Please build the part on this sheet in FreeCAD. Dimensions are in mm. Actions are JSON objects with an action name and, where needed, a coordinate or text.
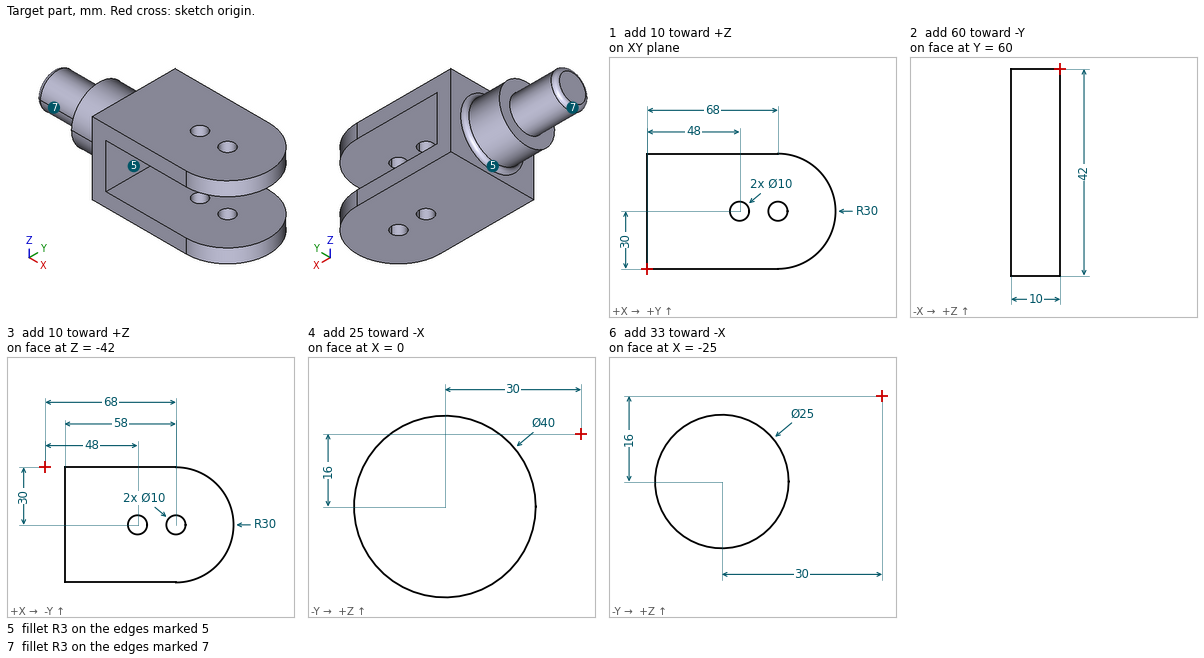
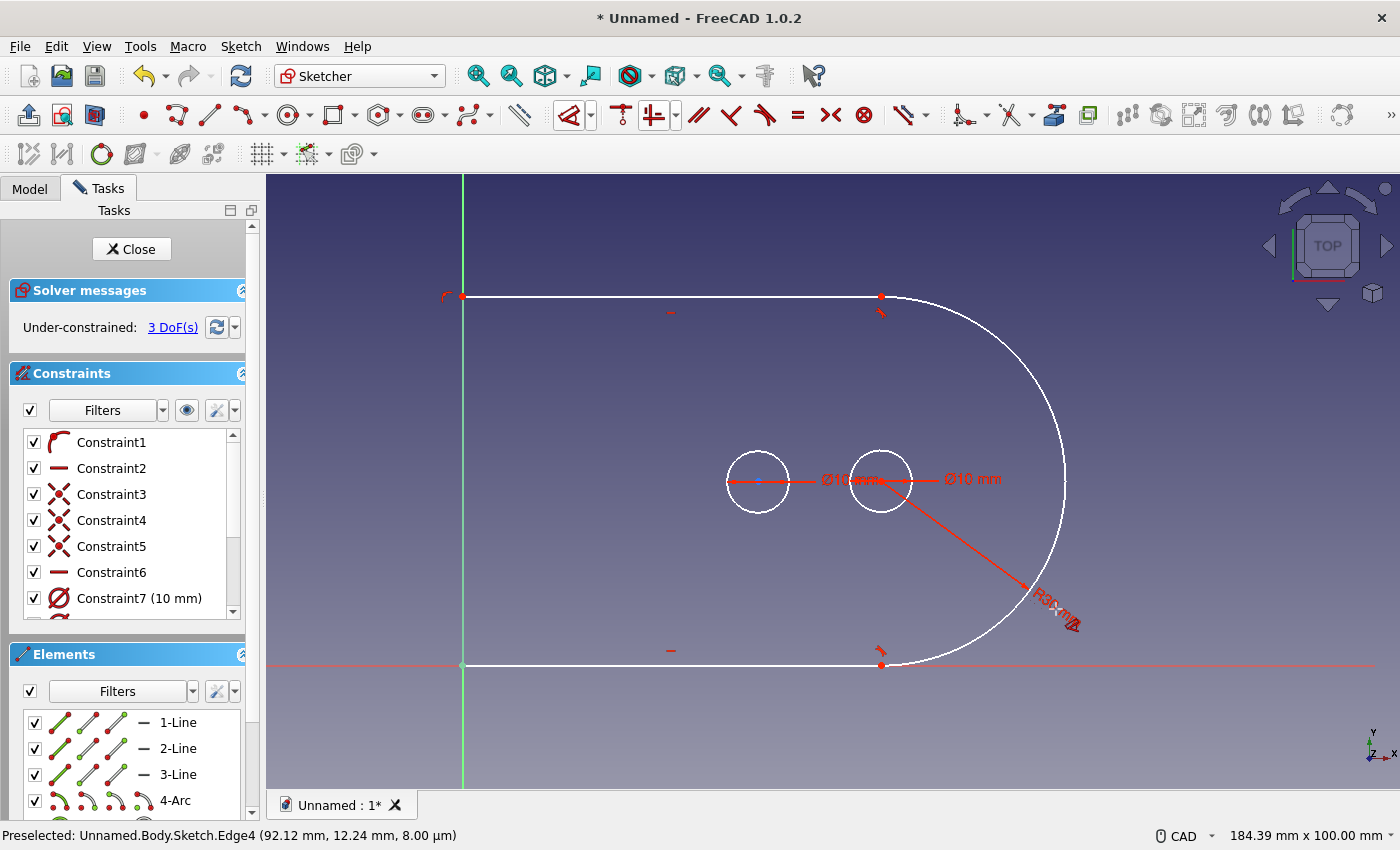
{"action": "left_click", "coordinate": [756, 297]}
{"action": "left_click", "coordinate": [672, 263]}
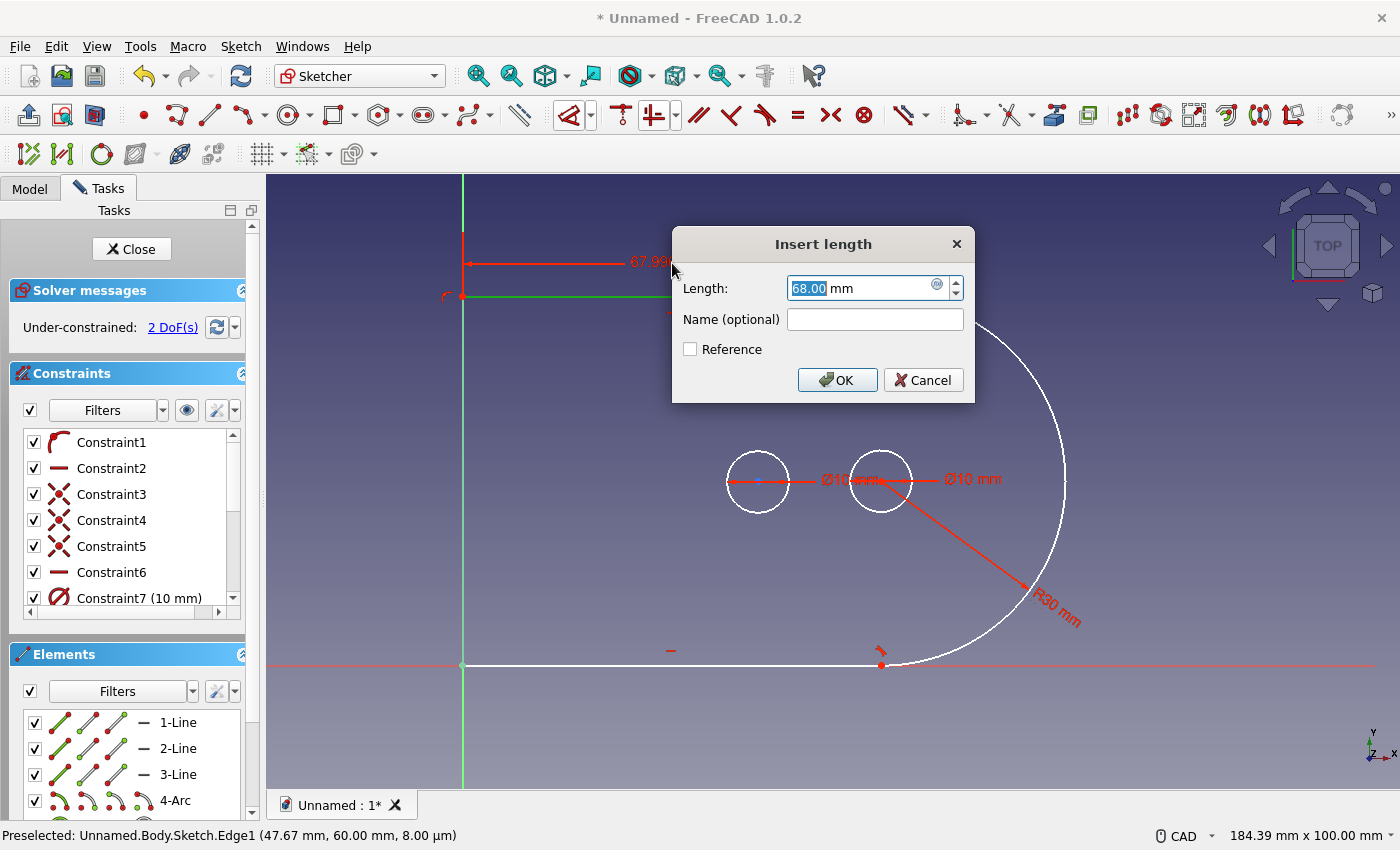
{"action": "type", "text": "68"}
{"action": "key", "text": "Return"}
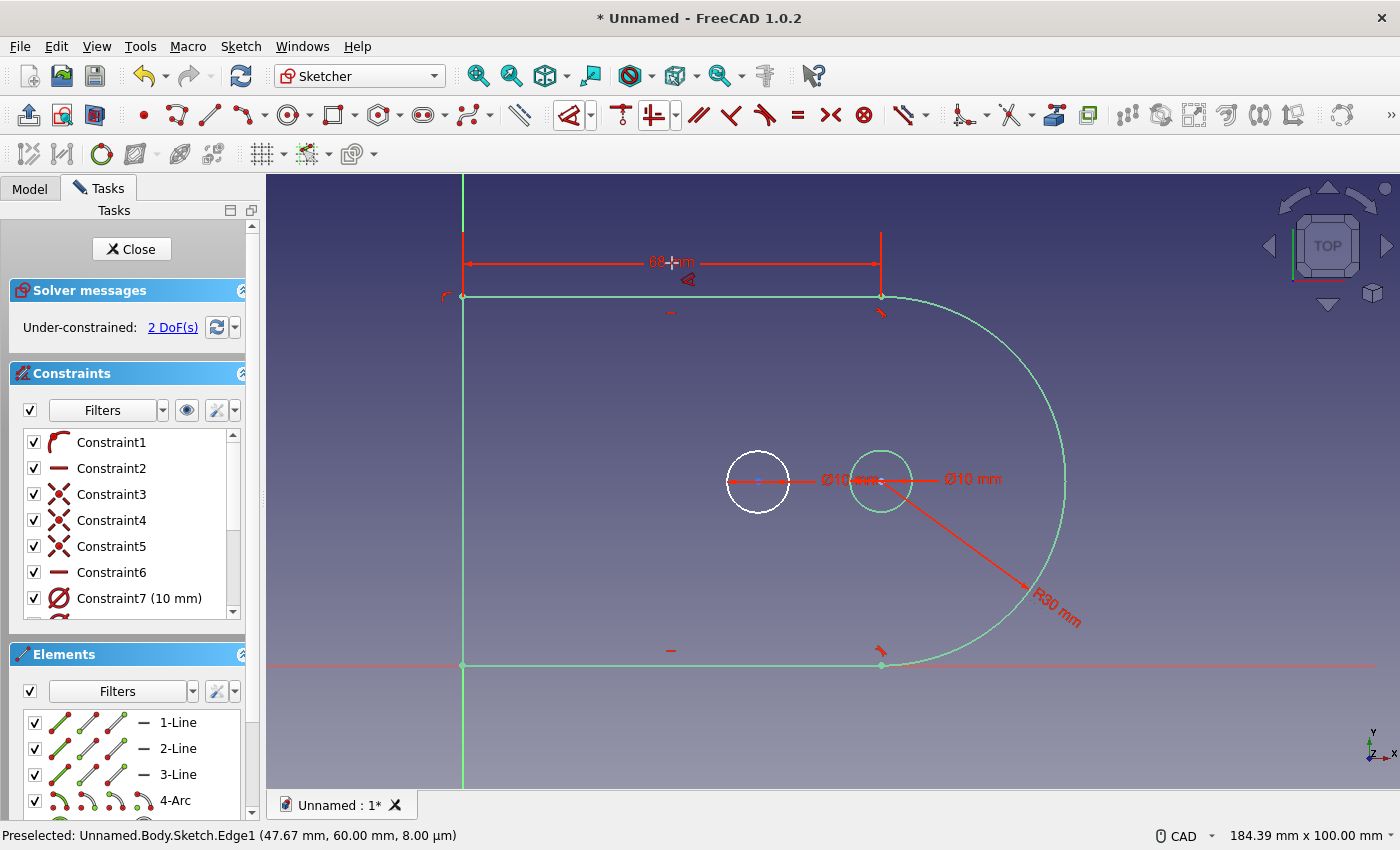
{"action": "left_click", "coordinate": [758, 482]}
{"action": "left_click", "coordinate": [610, 700]}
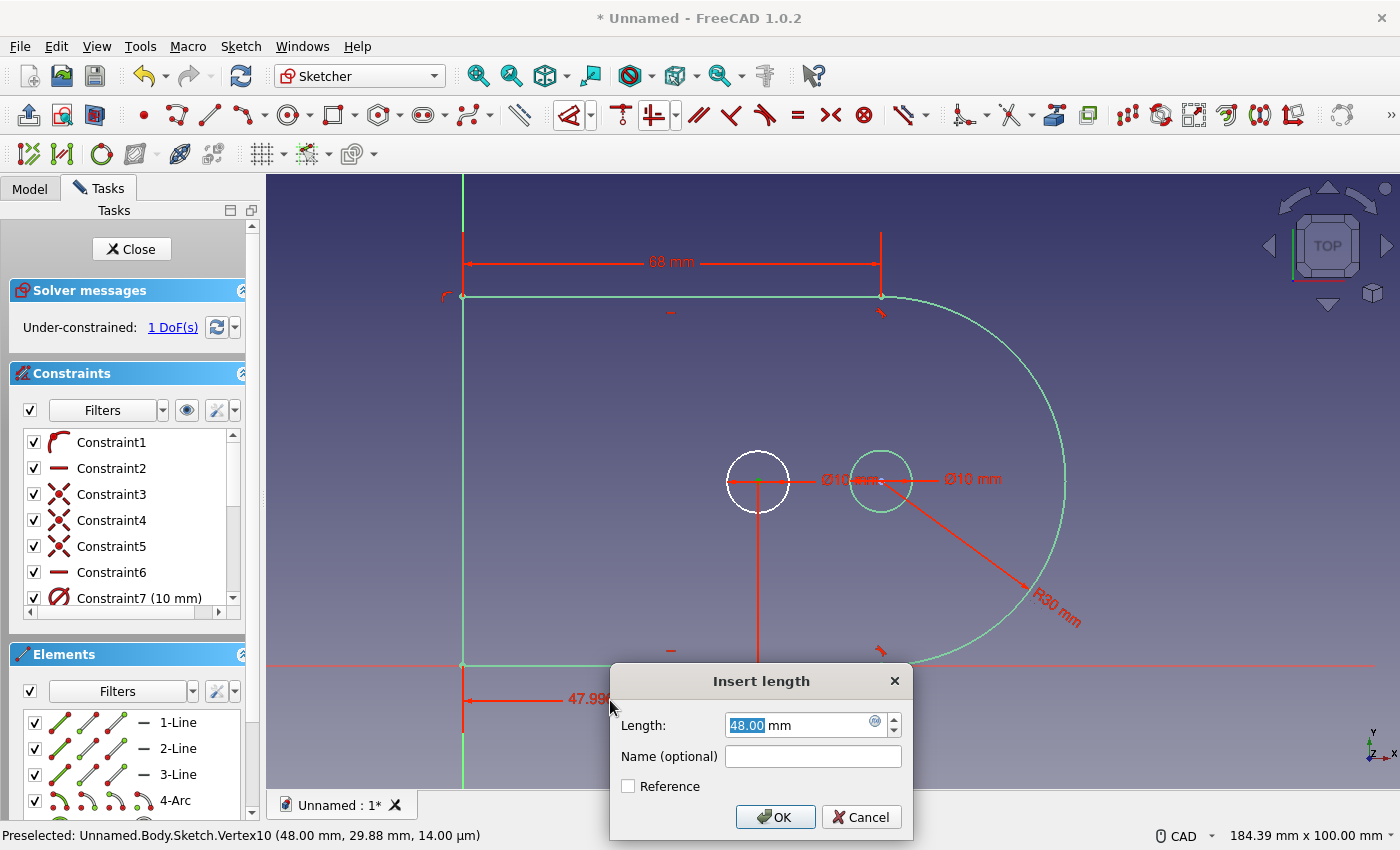
{"action": "type", "text": "48"}
{"action": "key", "text": "Return"}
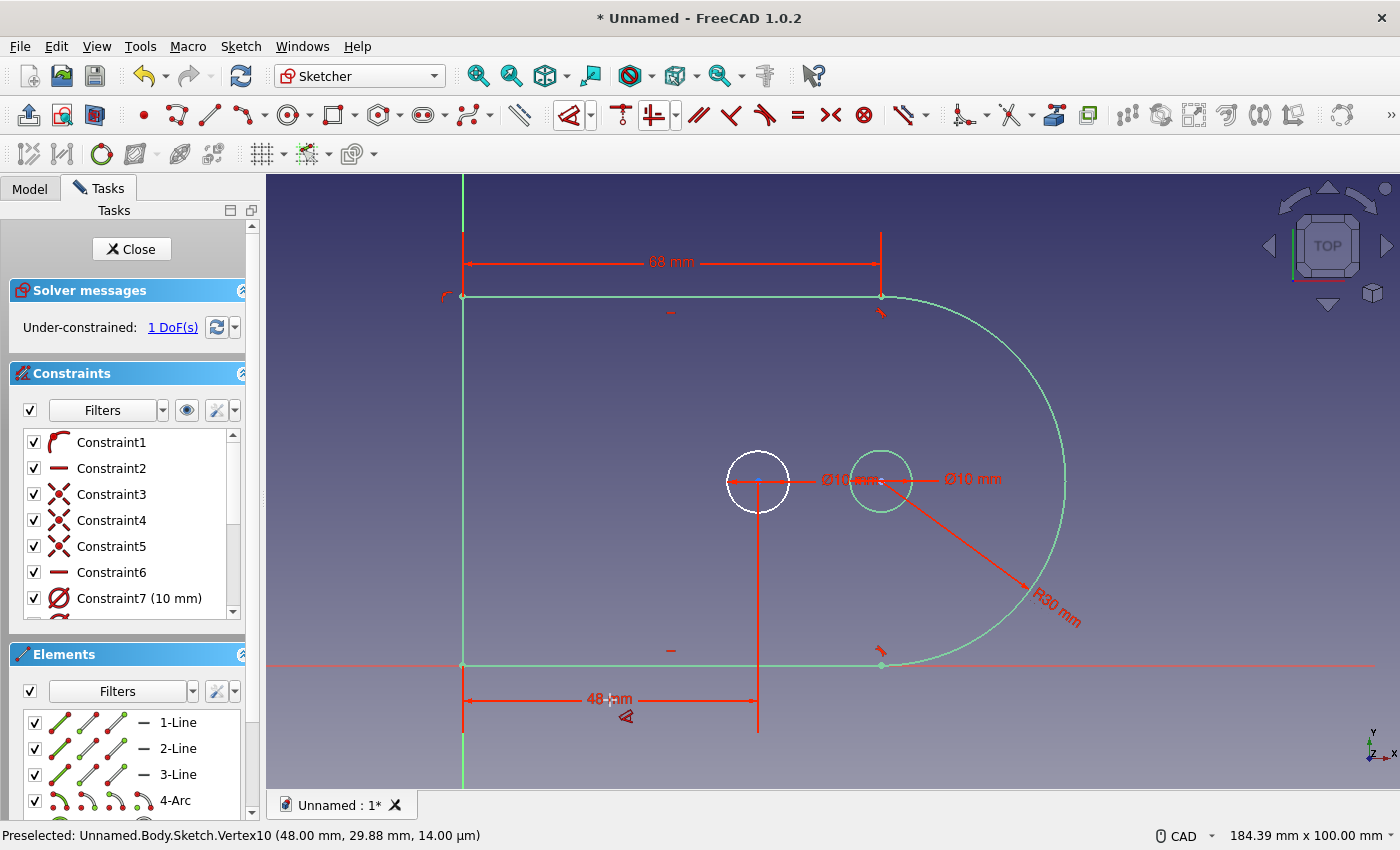
{"action": "left_click", "coordinate": [758, 482]}
{"action": "left_click", "coordinate": [429, 574]}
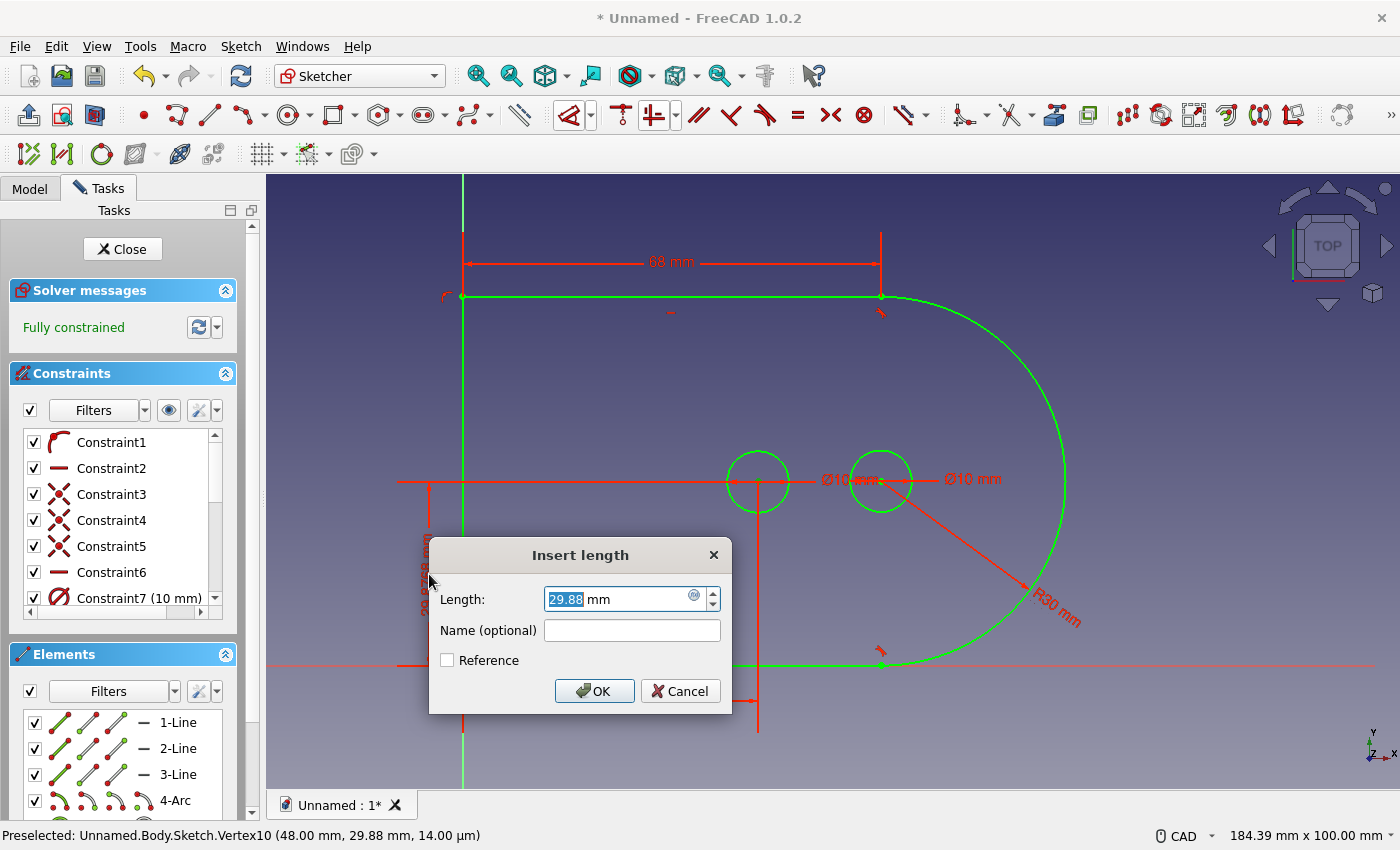
{"action": "type", "text": "30"}
{"action": "key", "text": "Return"}
{"action": "key", "text": "Escape"}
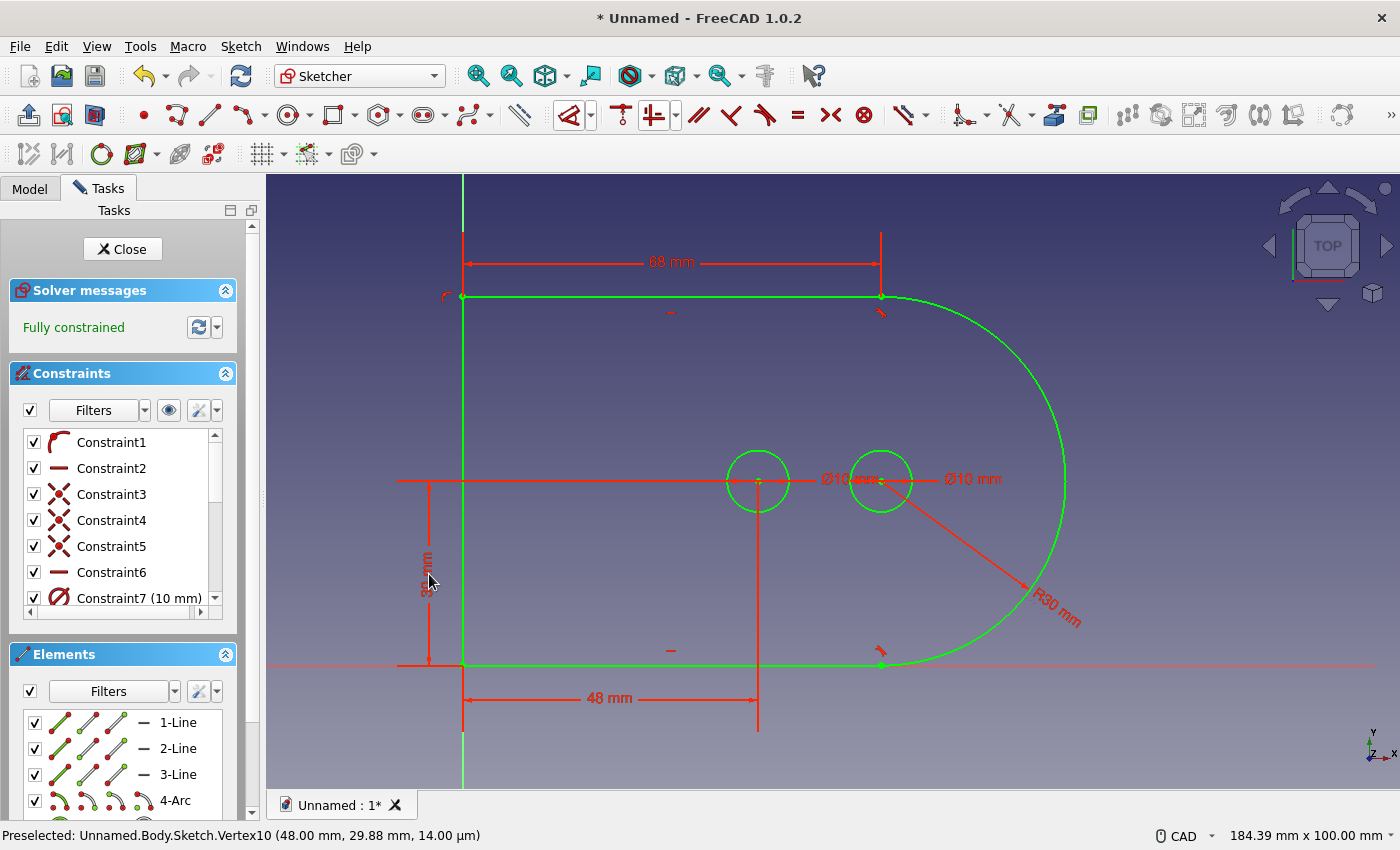
{"action": "left_click", "coordinate": [123, 249]}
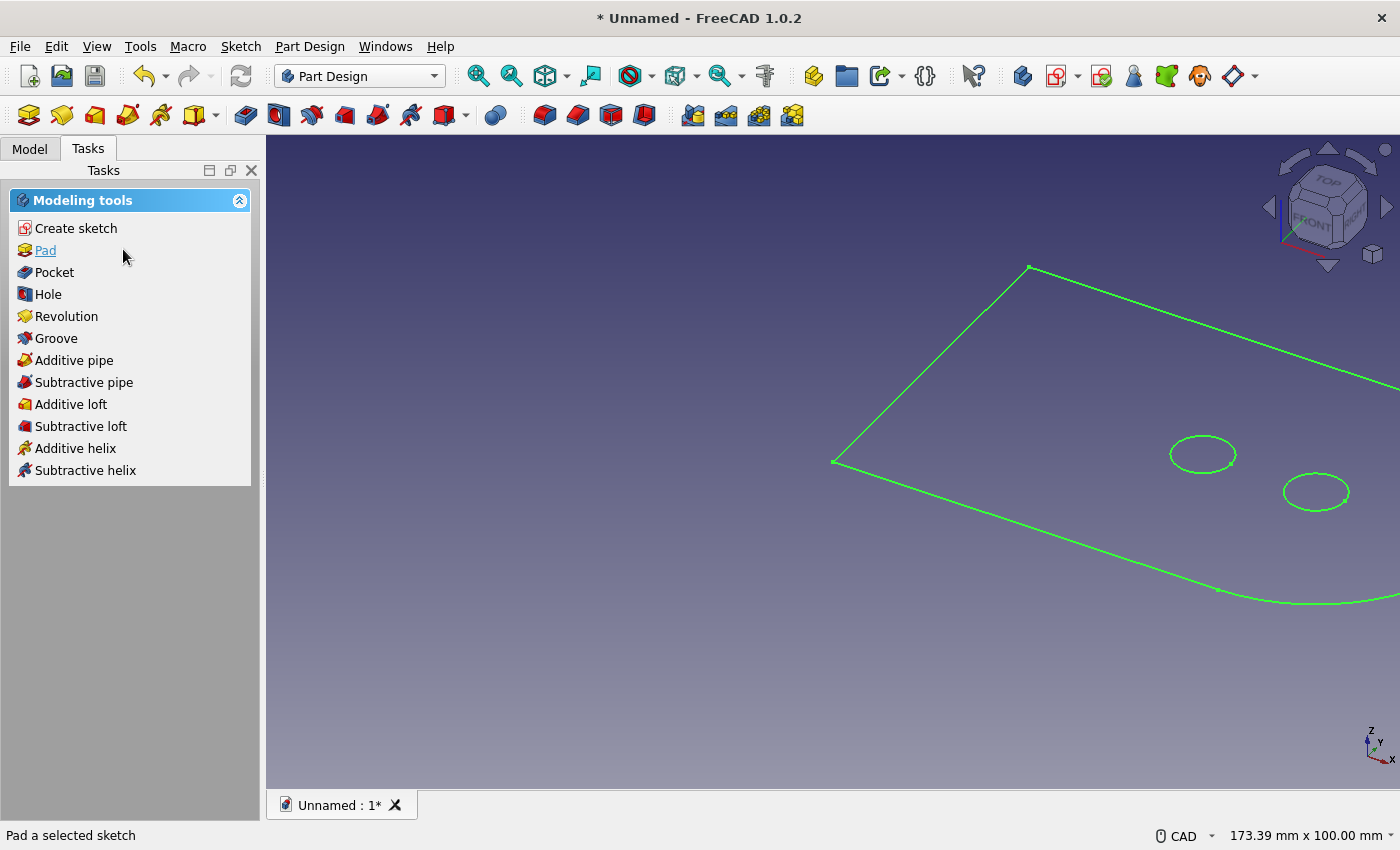
{"action": "left_click", "coordinate": [29, 116]}